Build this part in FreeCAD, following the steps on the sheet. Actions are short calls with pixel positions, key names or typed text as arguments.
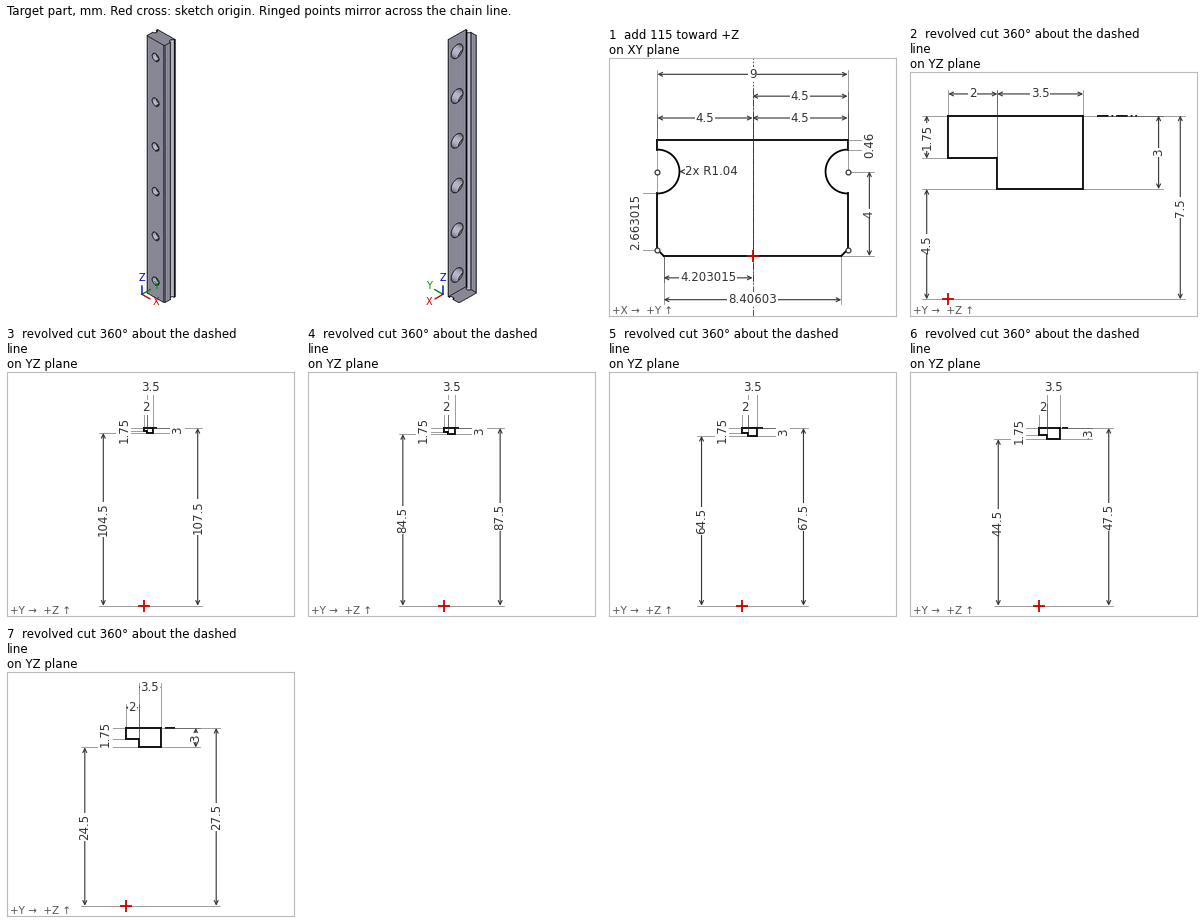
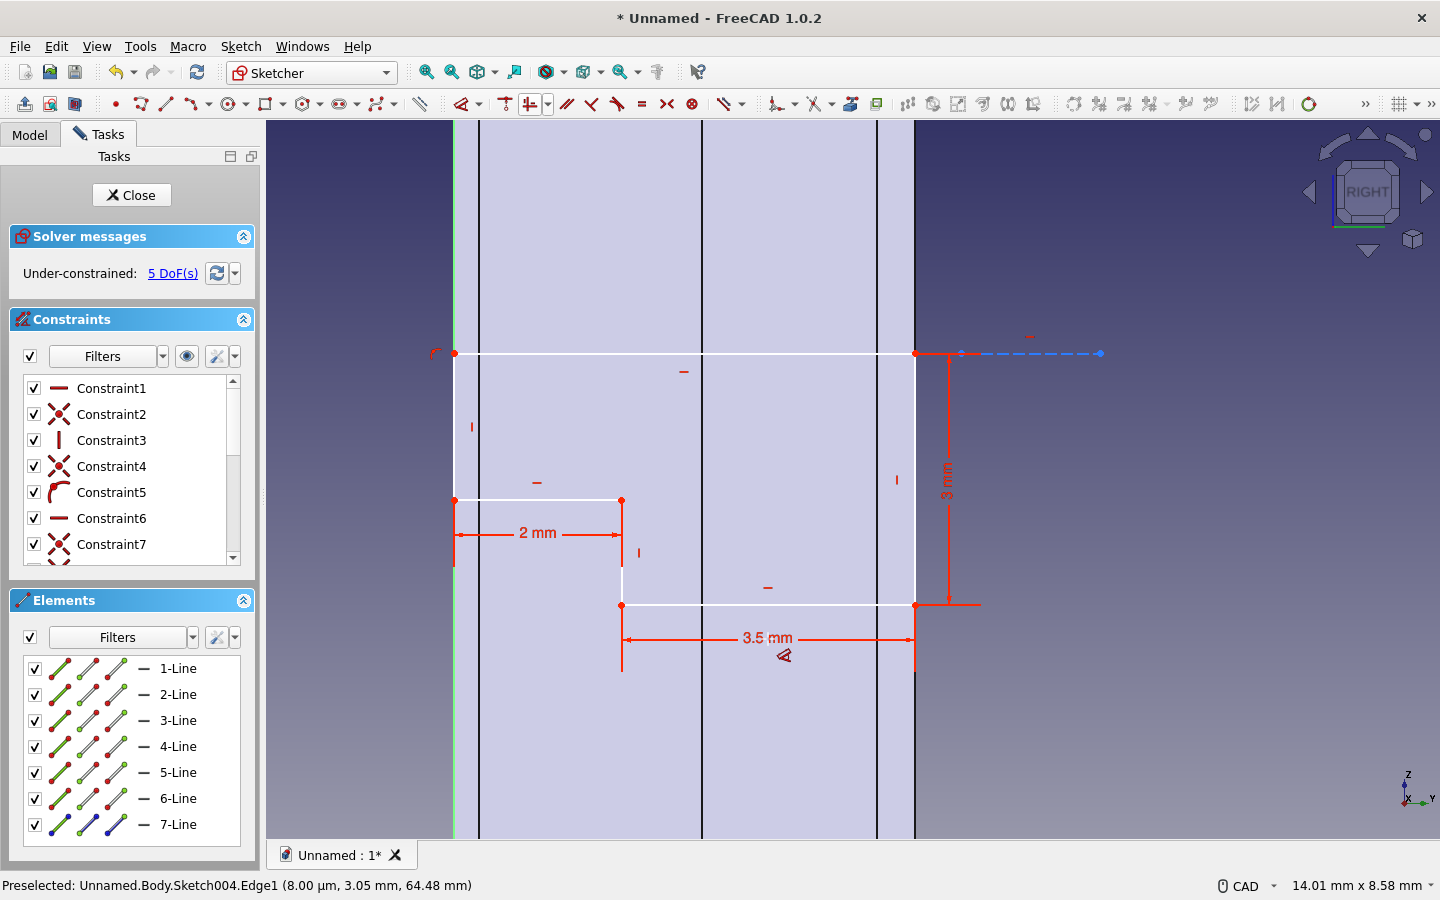
click(454, 398)
click(420, 427)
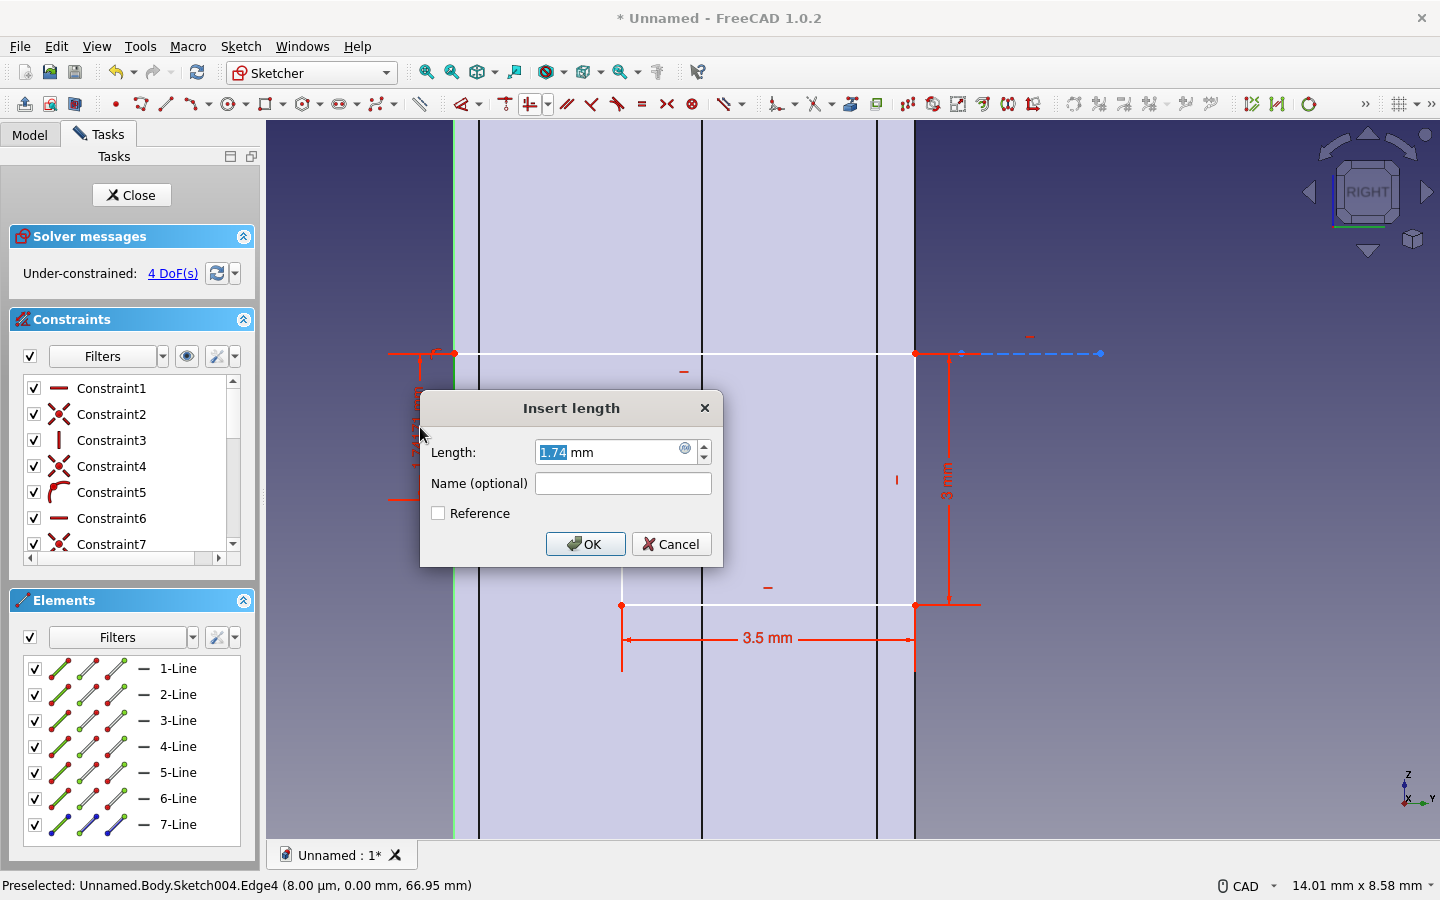
text(1.75)
key(Return)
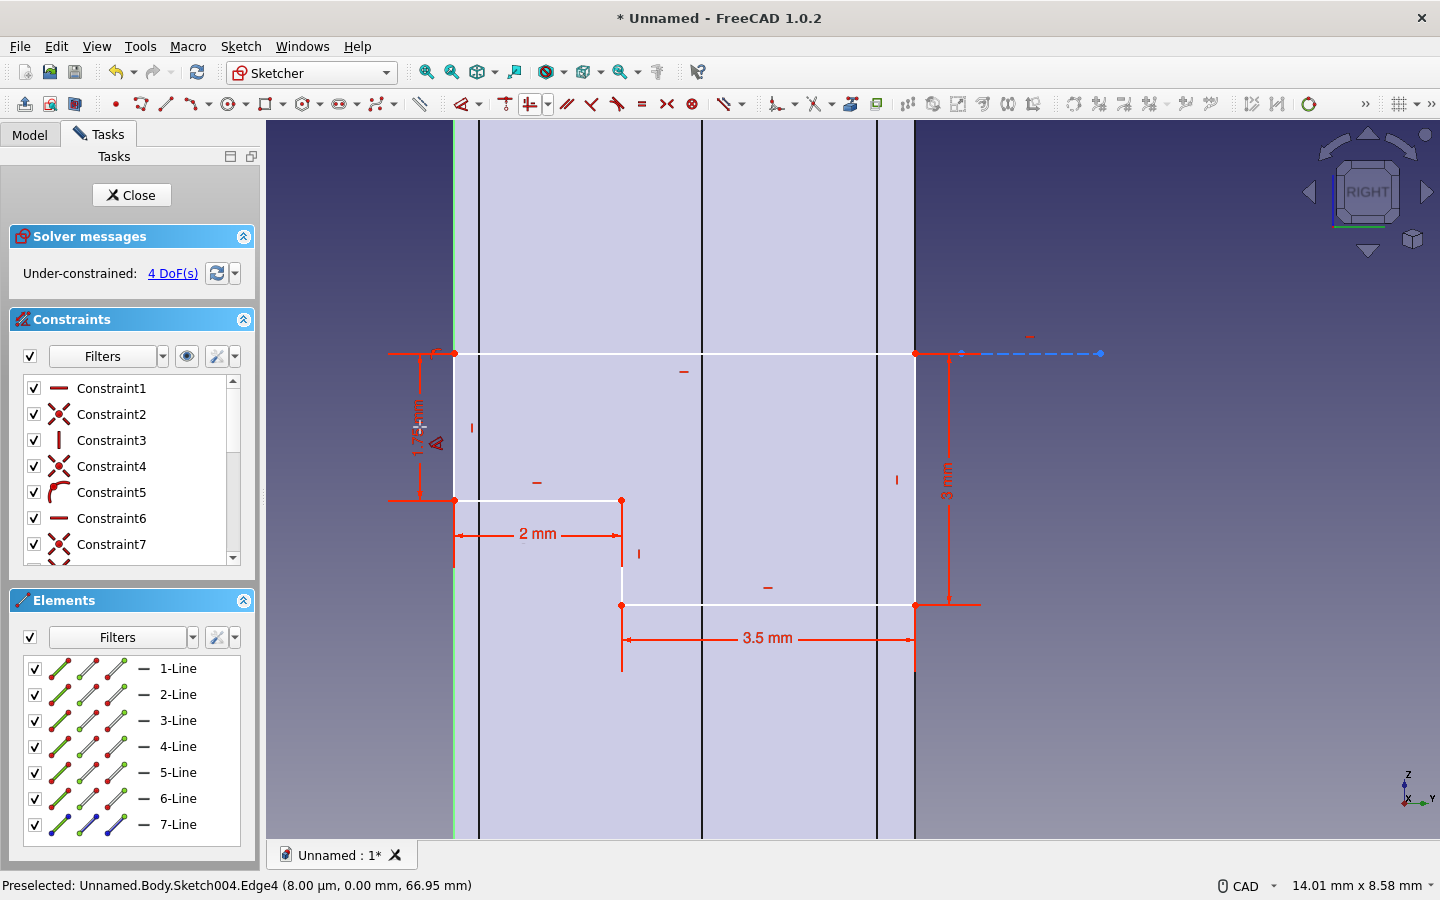
click(622, 605)
click(420, 708)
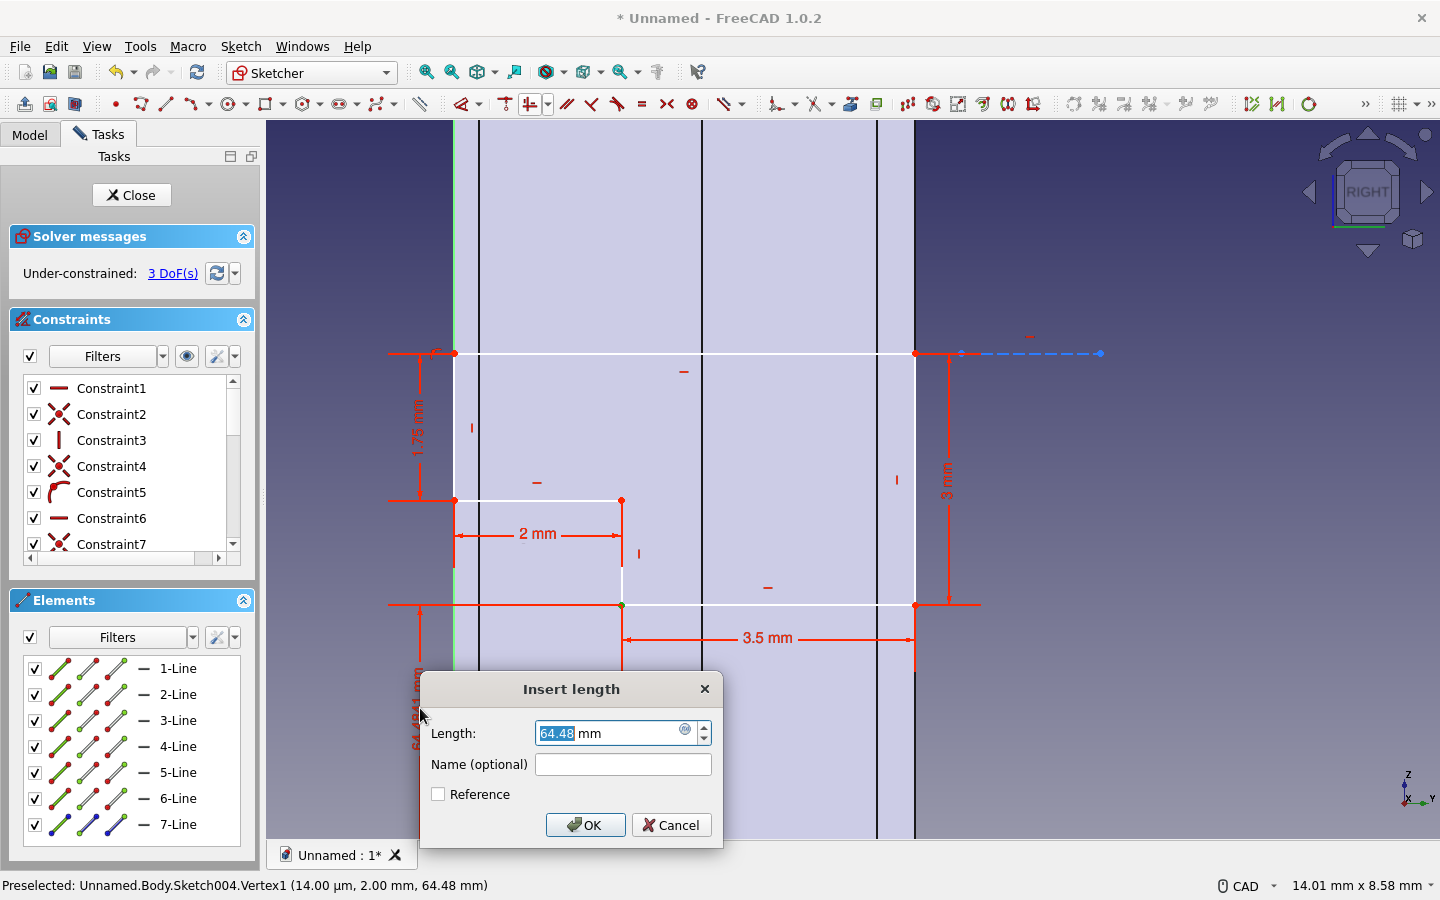
text(64.5)
key(Return)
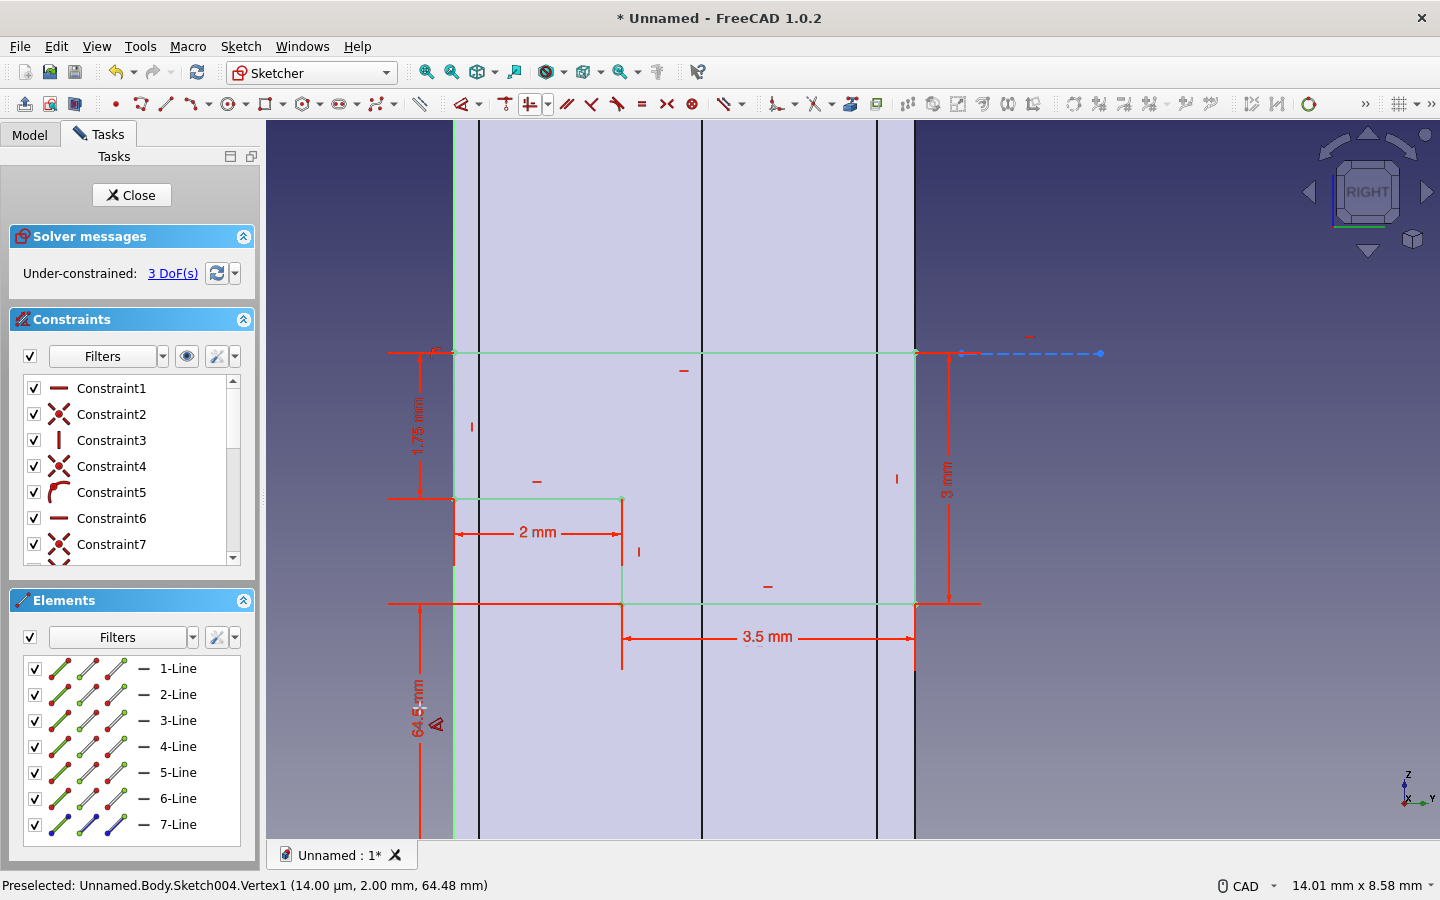
click(961, 354)
click(420, 582)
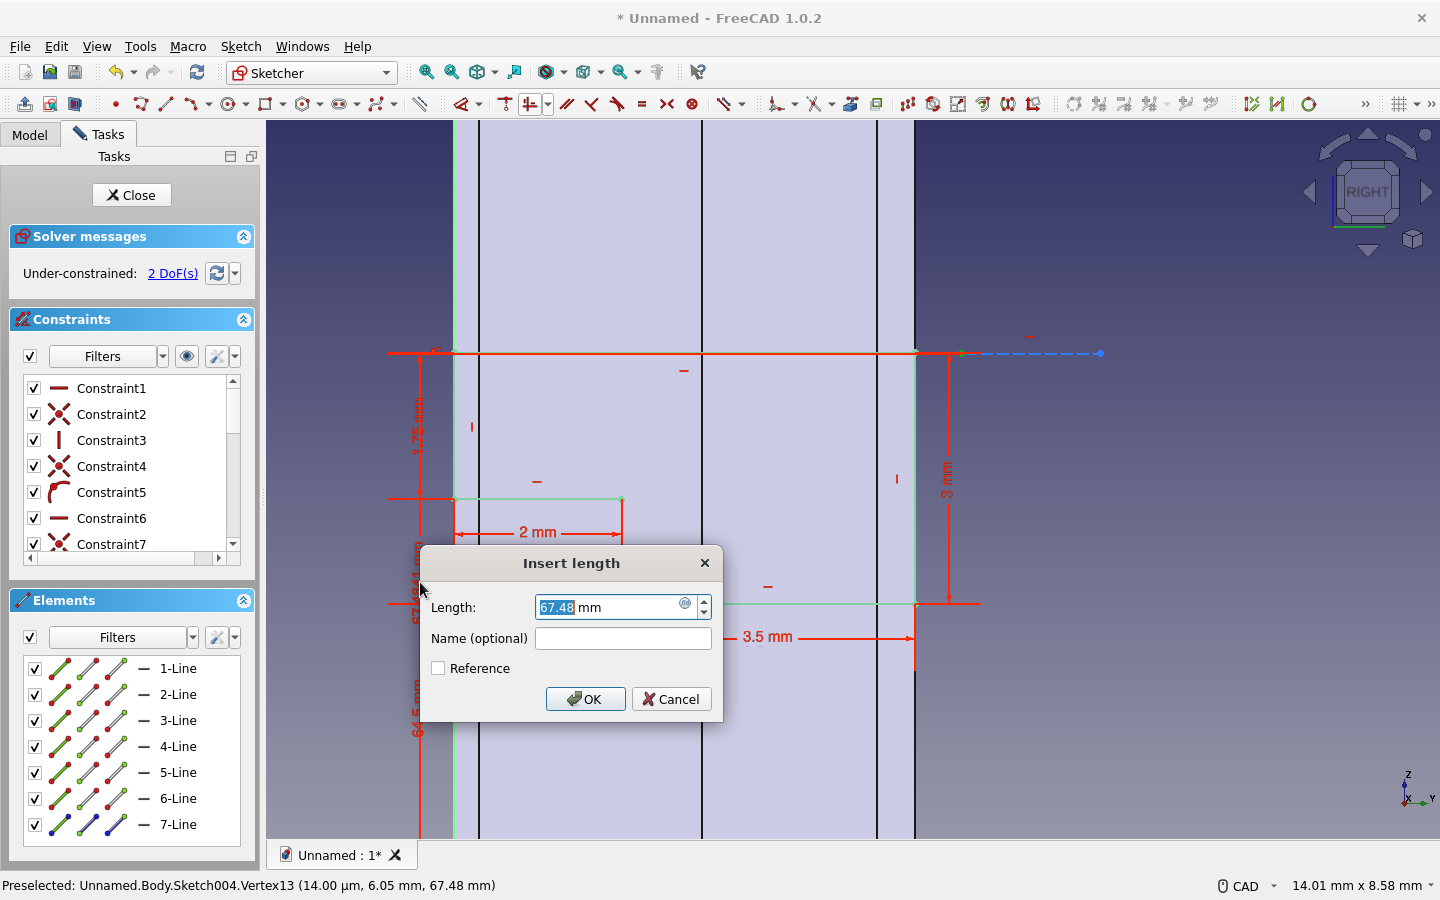
text(67.5)
key(Return)
key(Escape)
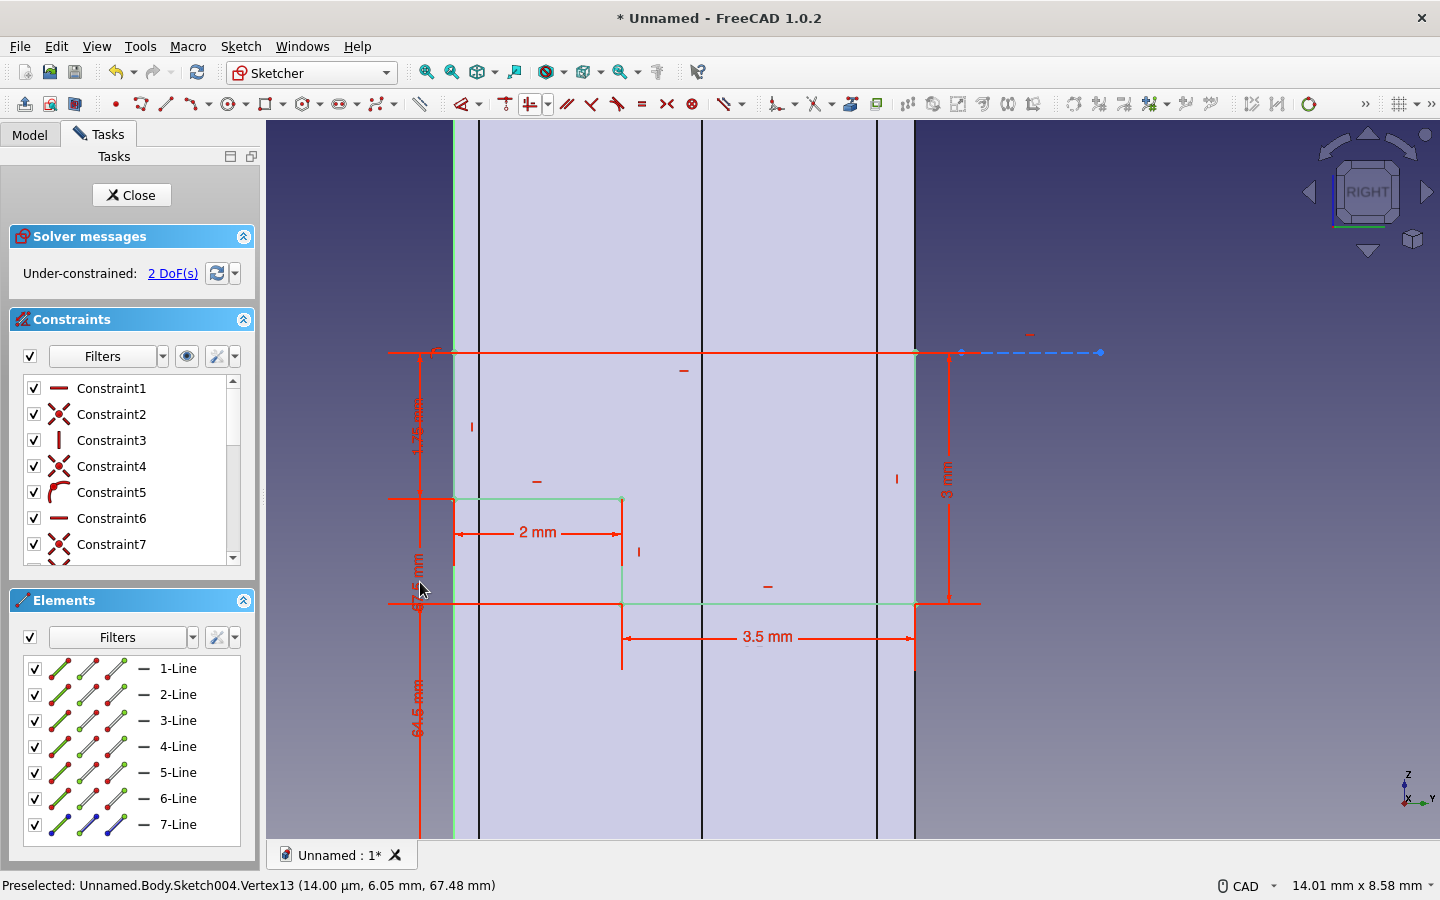
click(132, 195)